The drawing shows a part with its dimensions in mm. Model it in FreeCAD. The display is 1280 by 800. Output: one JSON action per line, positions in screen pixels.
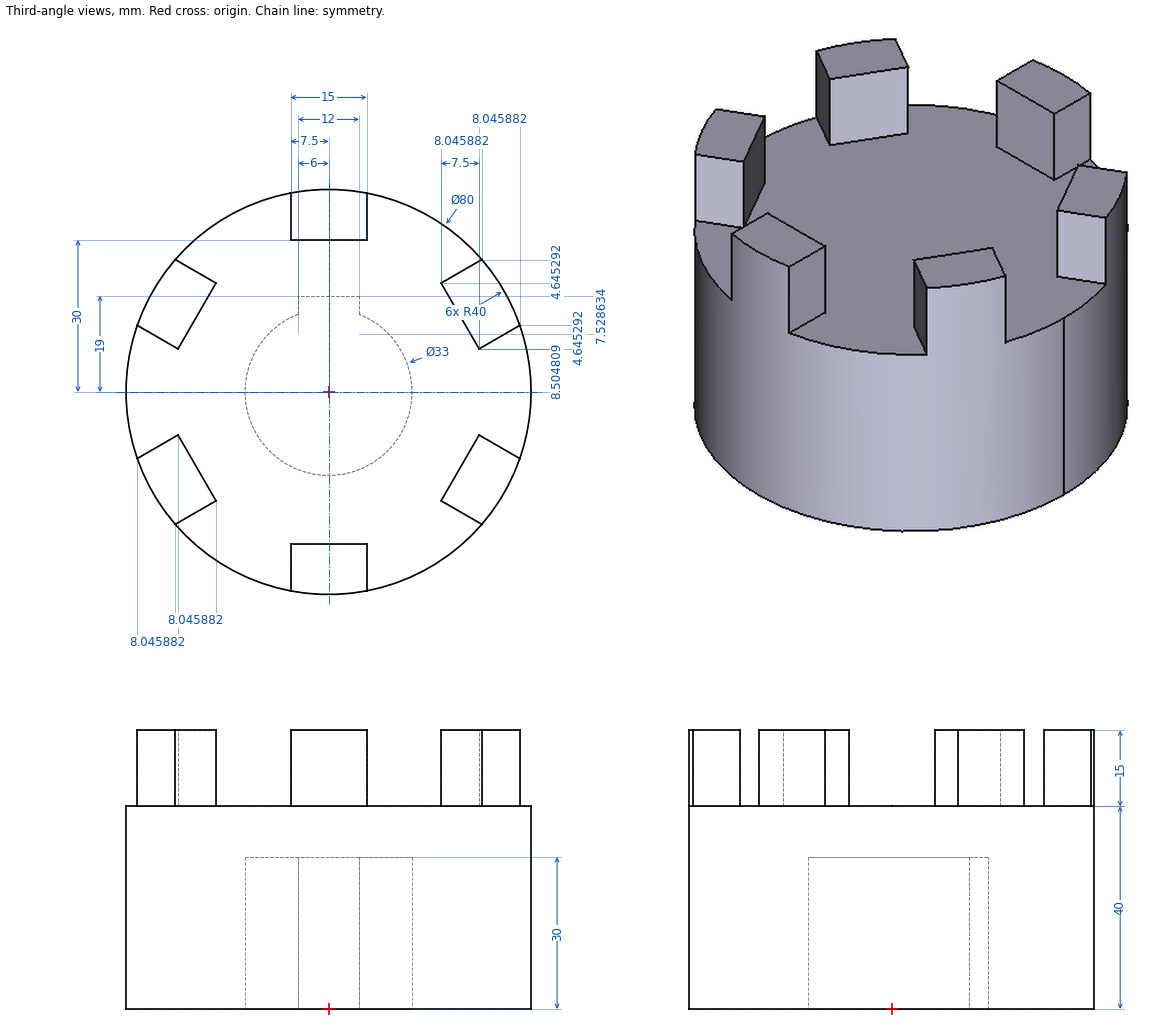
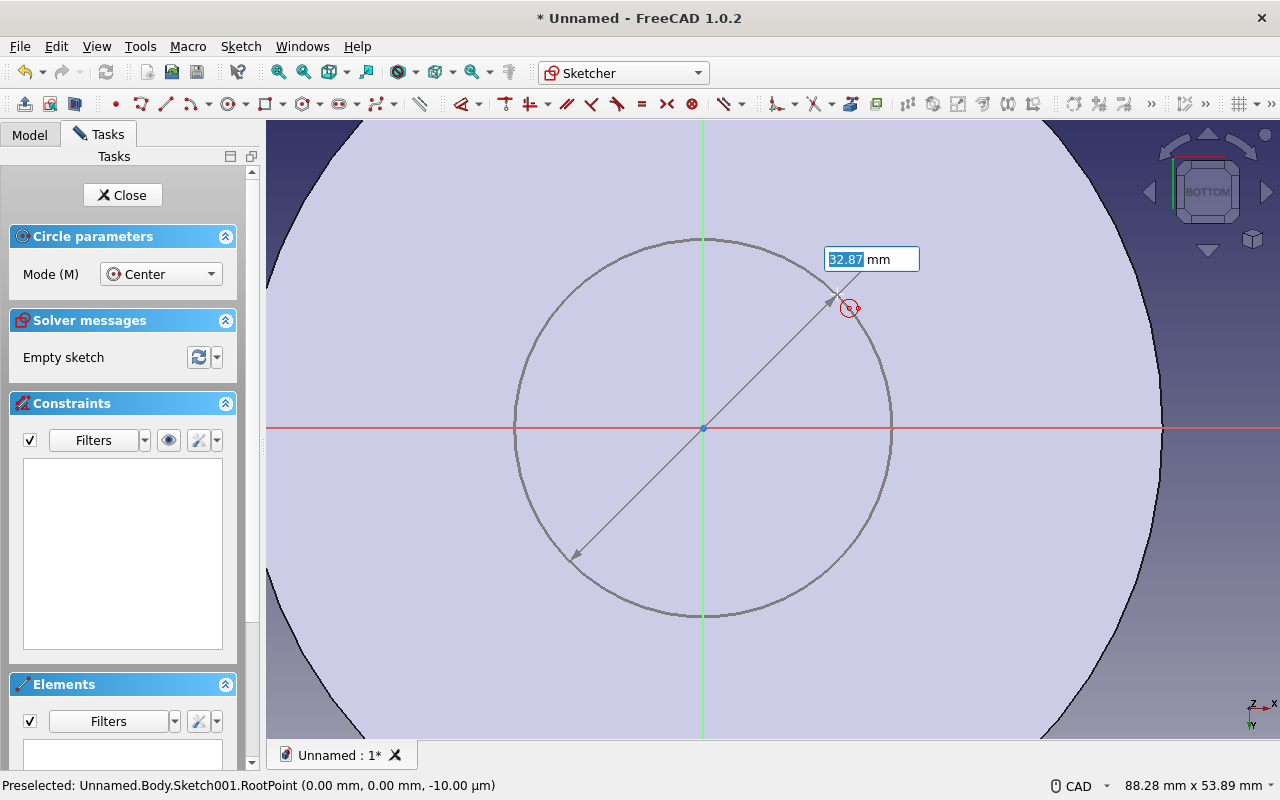
{"action": "type", "text": "33"}
{"action": "key", "text": "Return"}
{"action": "key", "text": "Escape"}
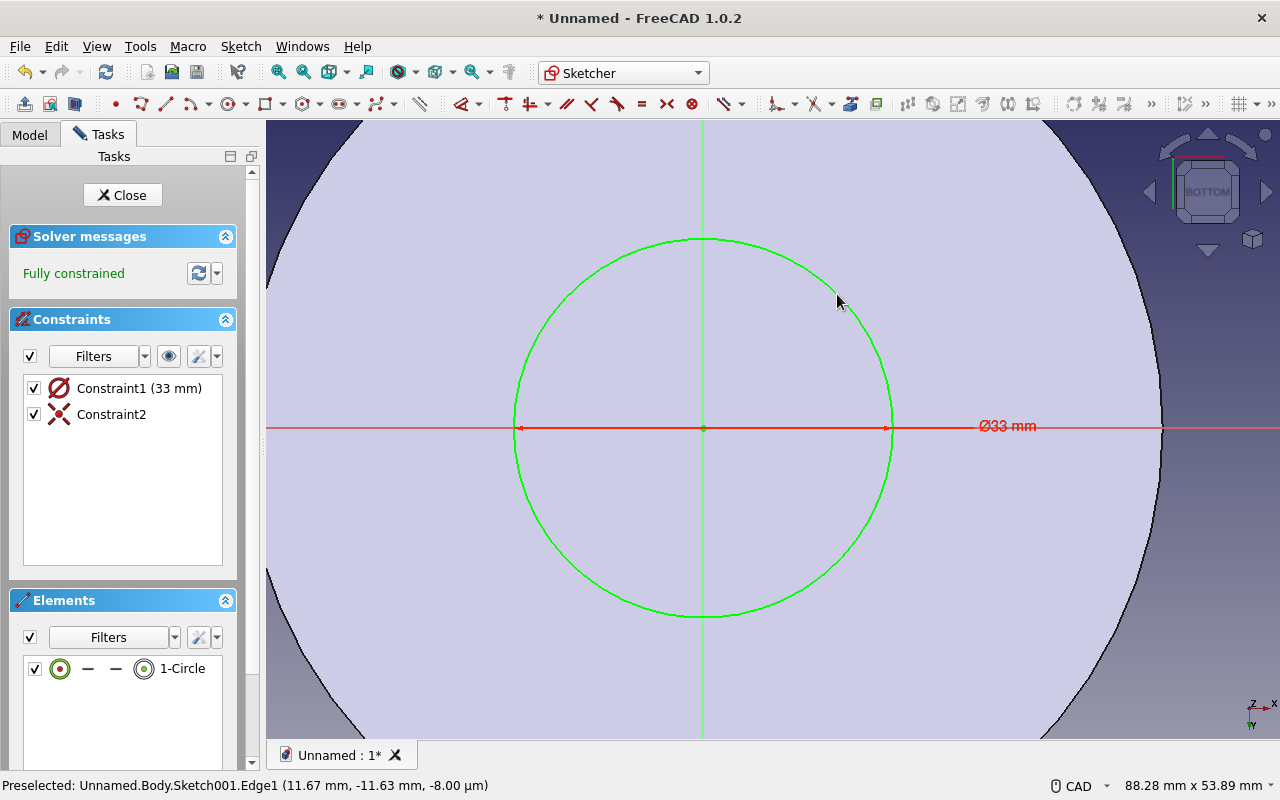
{"action": "left_click", "coordinate": [123, 195]}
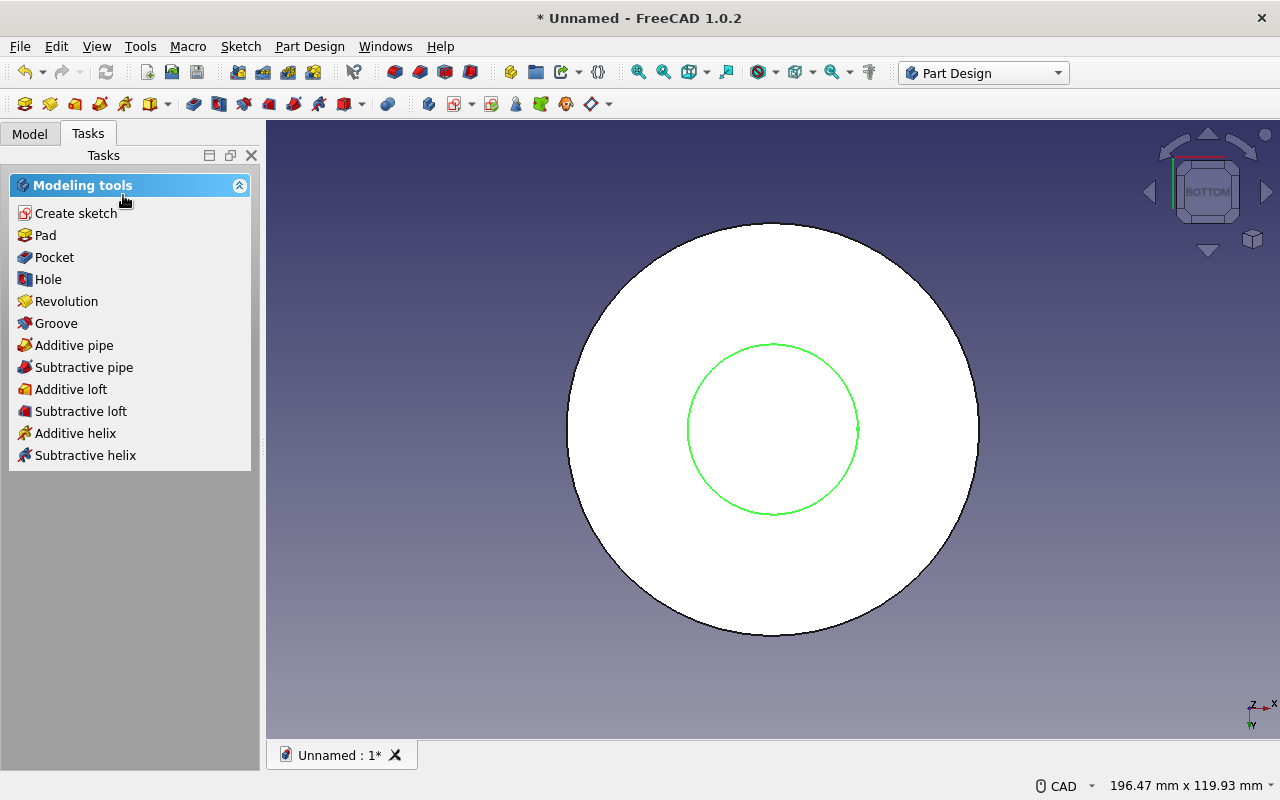
{"action": "left_click", "coordinate": [194, 104]}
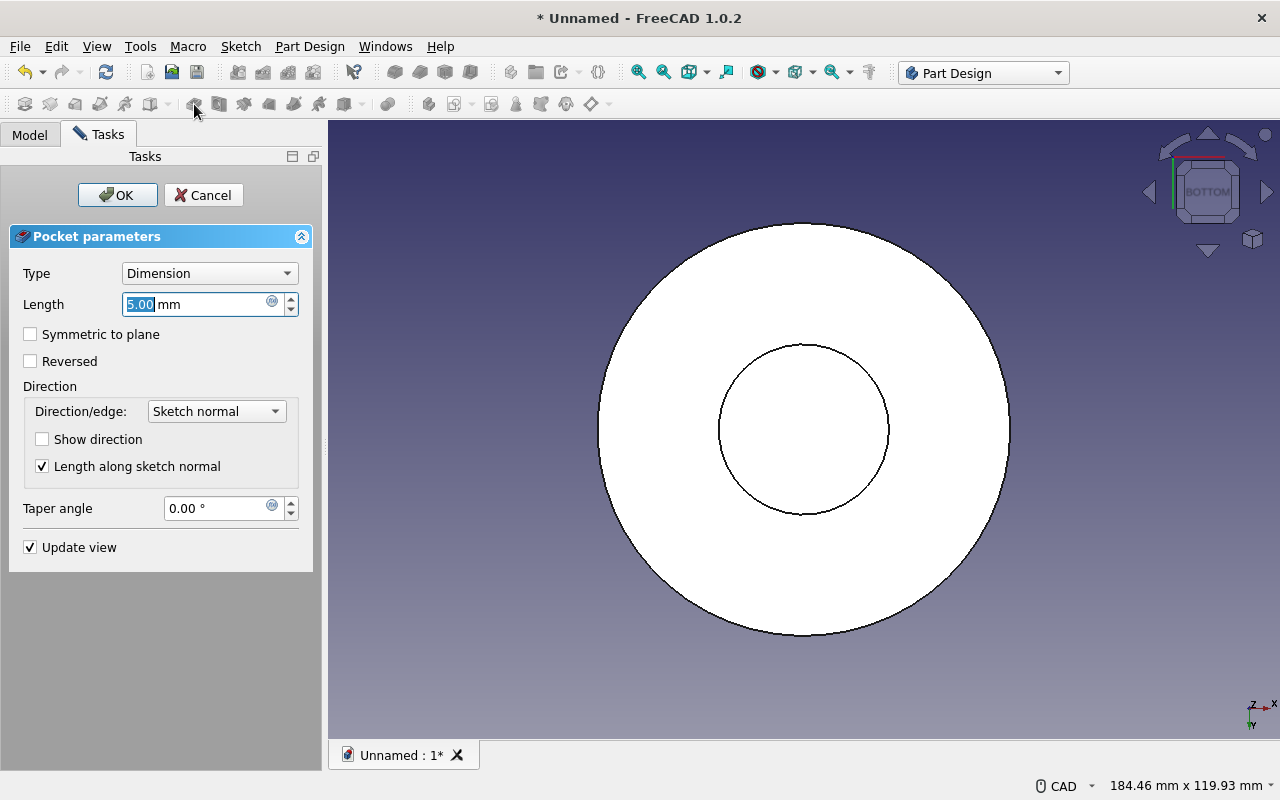
{"action": "type", "text": "30"}
{"action": "key", "text": "Tab"}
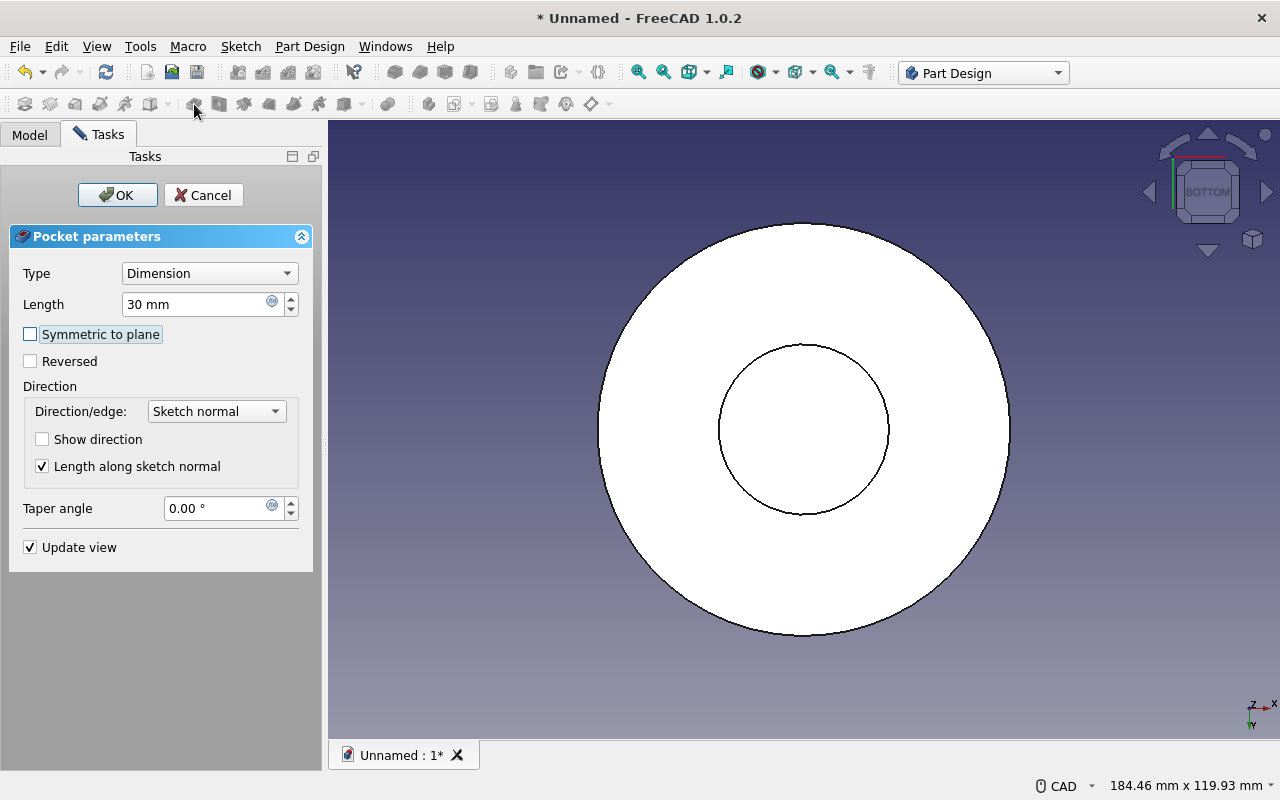
{"action": "left_click", "coordinate": [118, 195]}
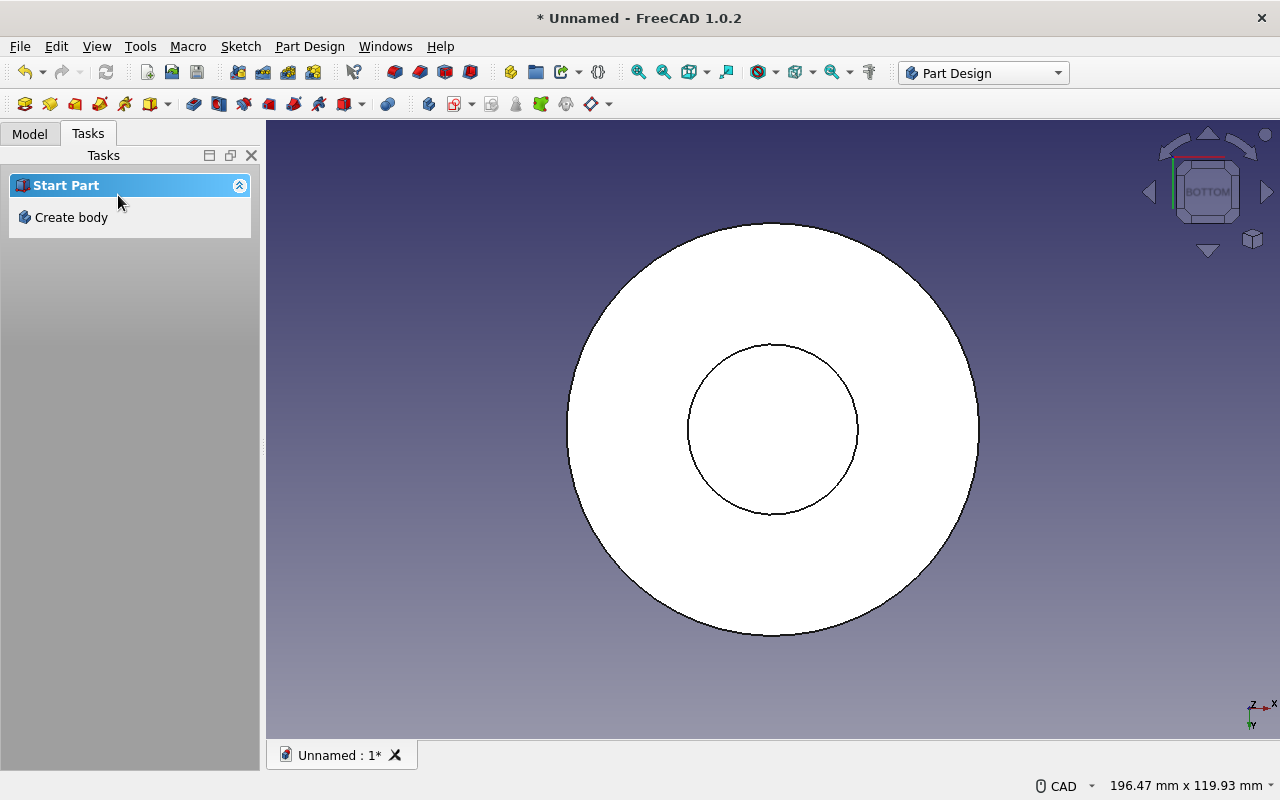
{"action": "key", "text": "0"}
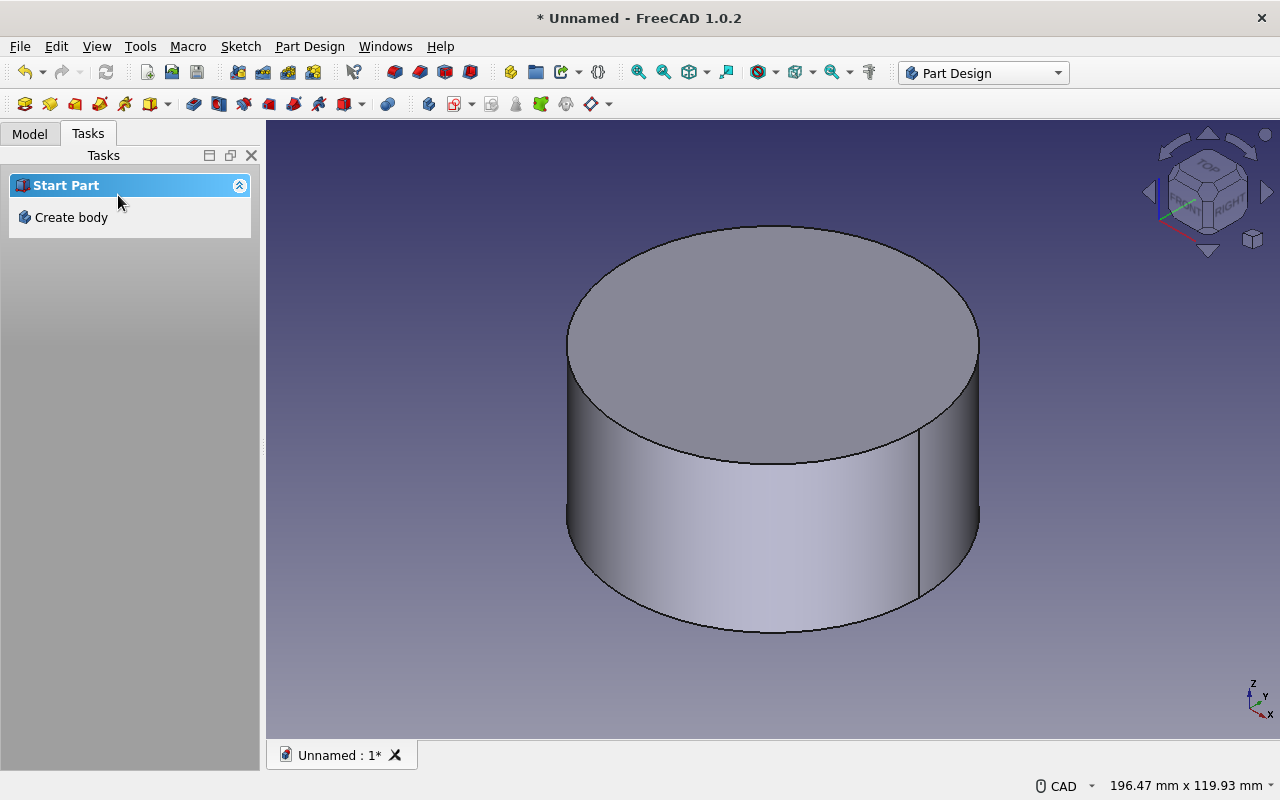
{"action": "left_click", "coordinate": [773, 344]}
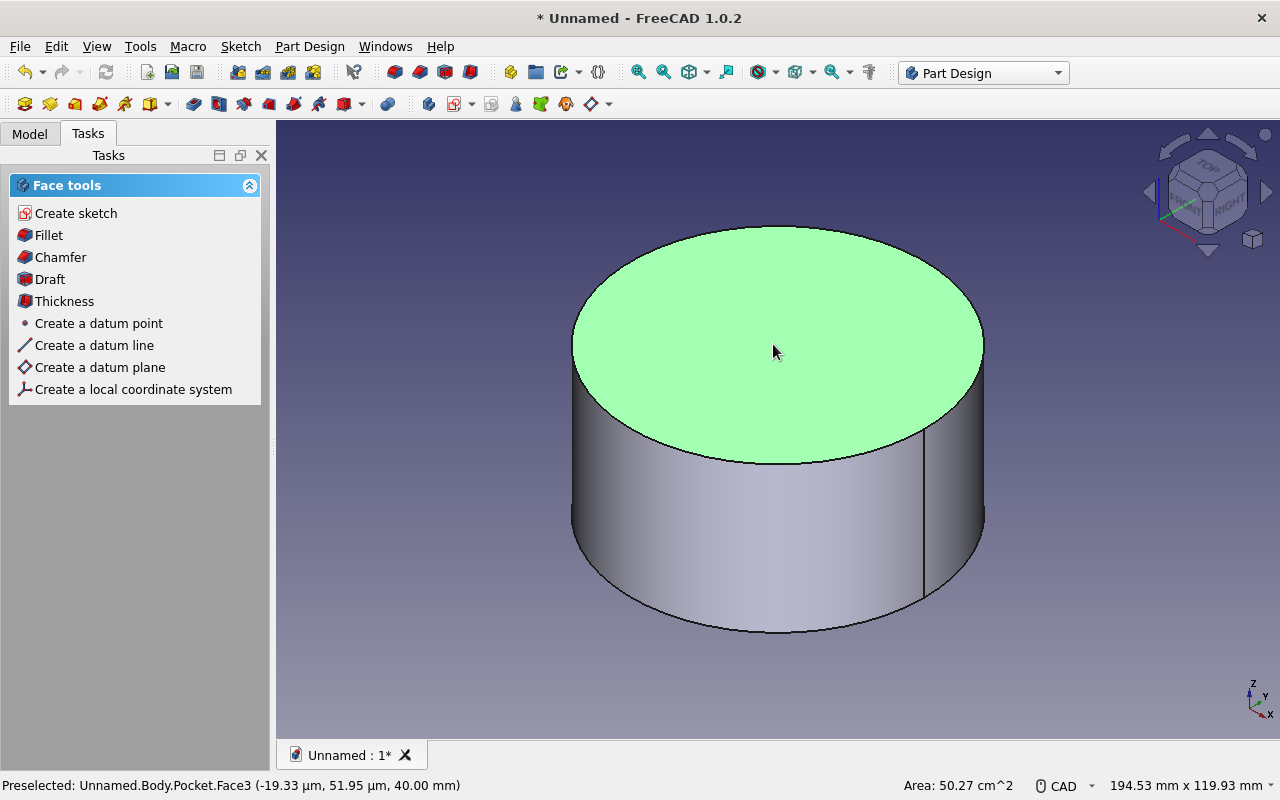
{"action": "left_click", "coordinate": [454, 104]}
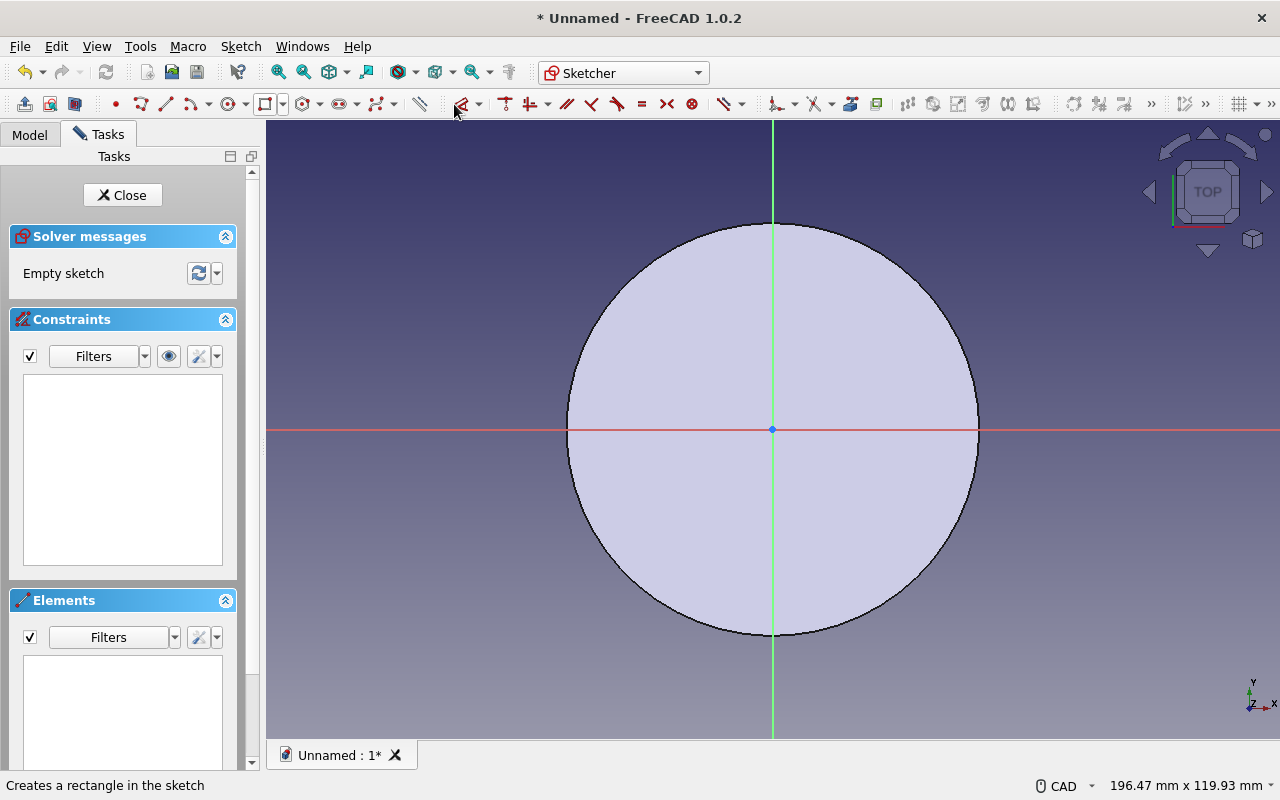
{"action": "key", "text": "g m"}